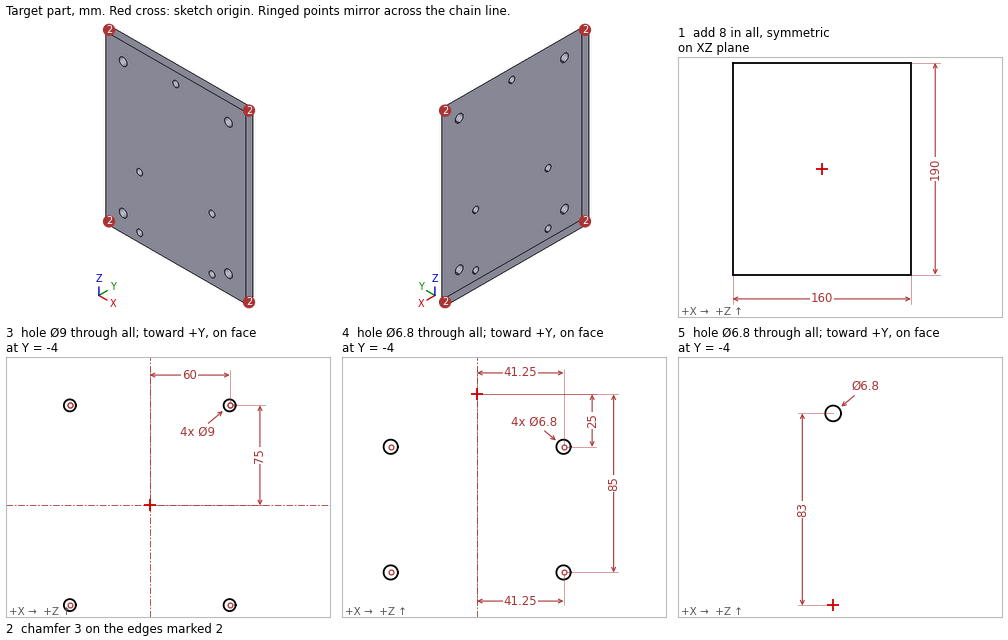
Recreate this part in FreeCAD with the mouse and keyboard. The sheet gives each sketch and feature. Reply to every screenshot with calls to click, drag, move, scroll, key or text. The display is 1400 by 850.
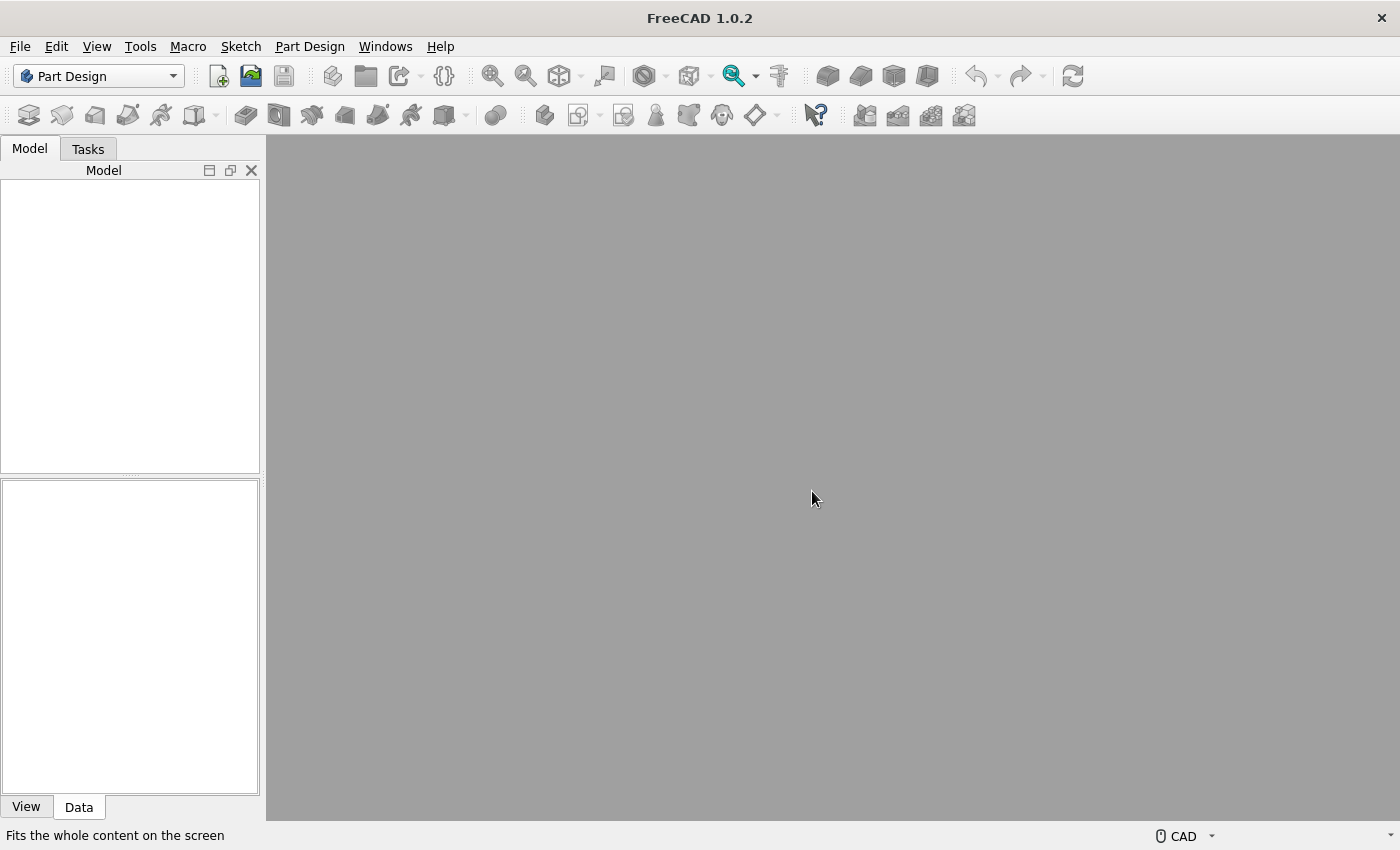
click(218, 76)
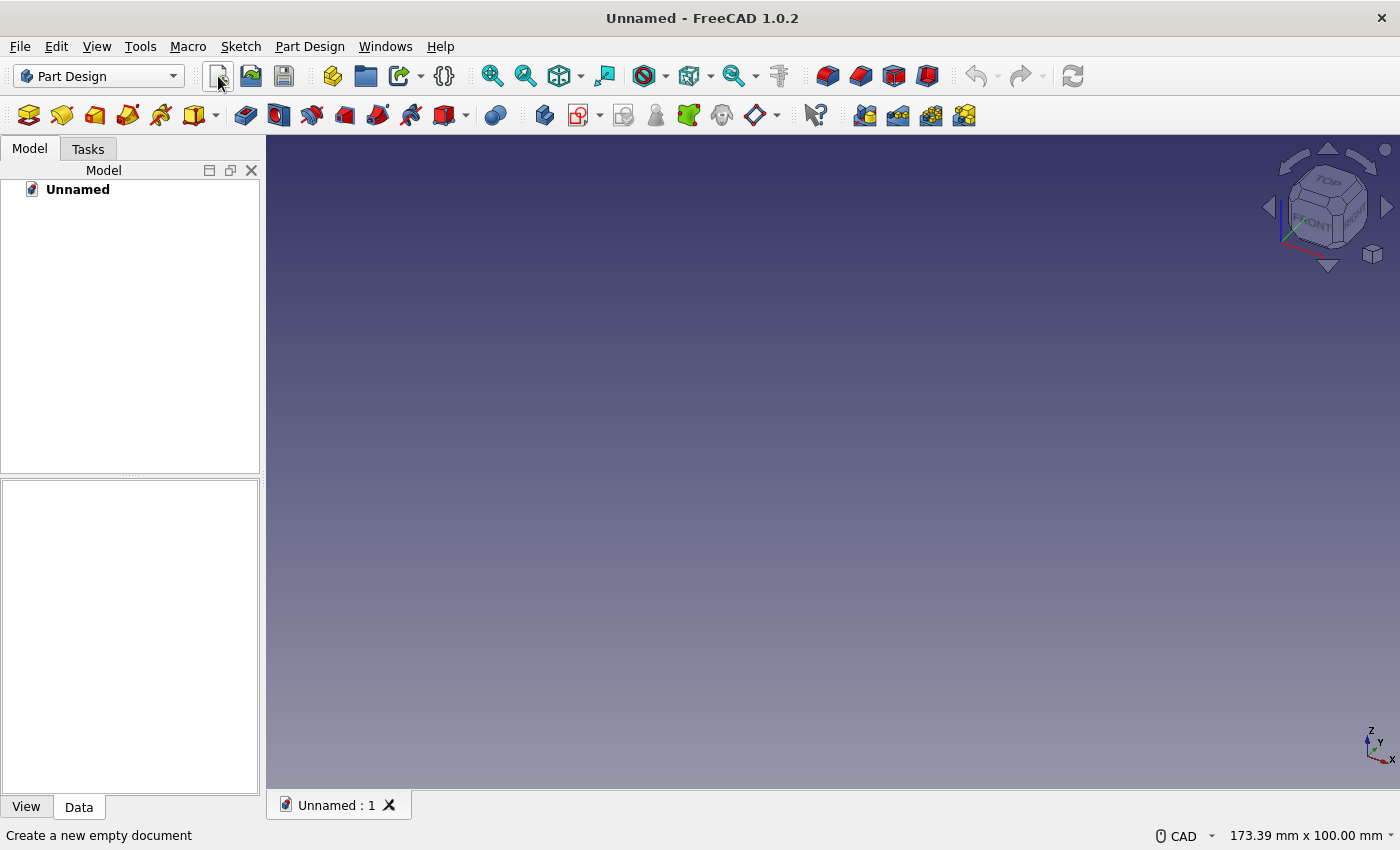
click(578, 116)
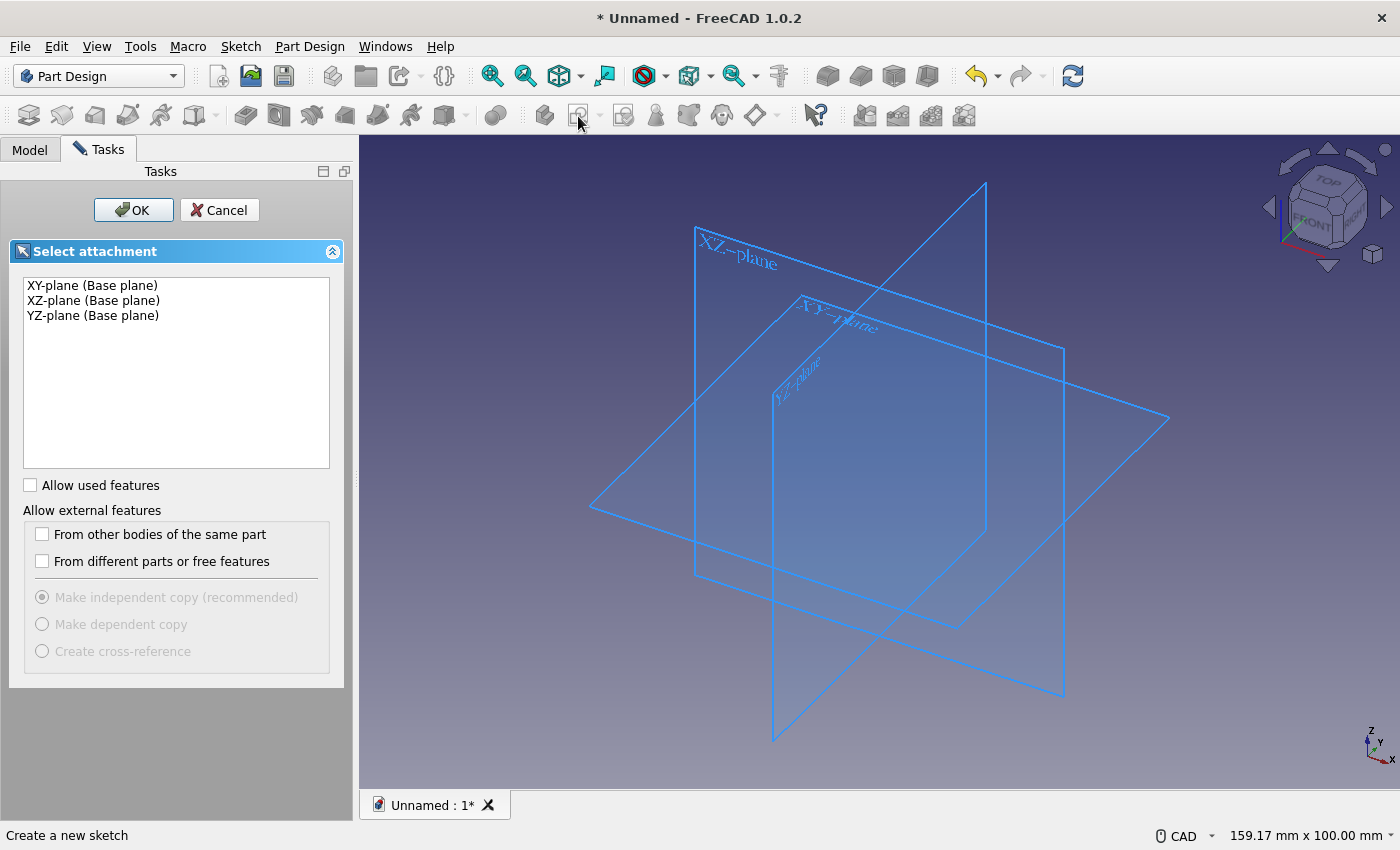
click(84, 300)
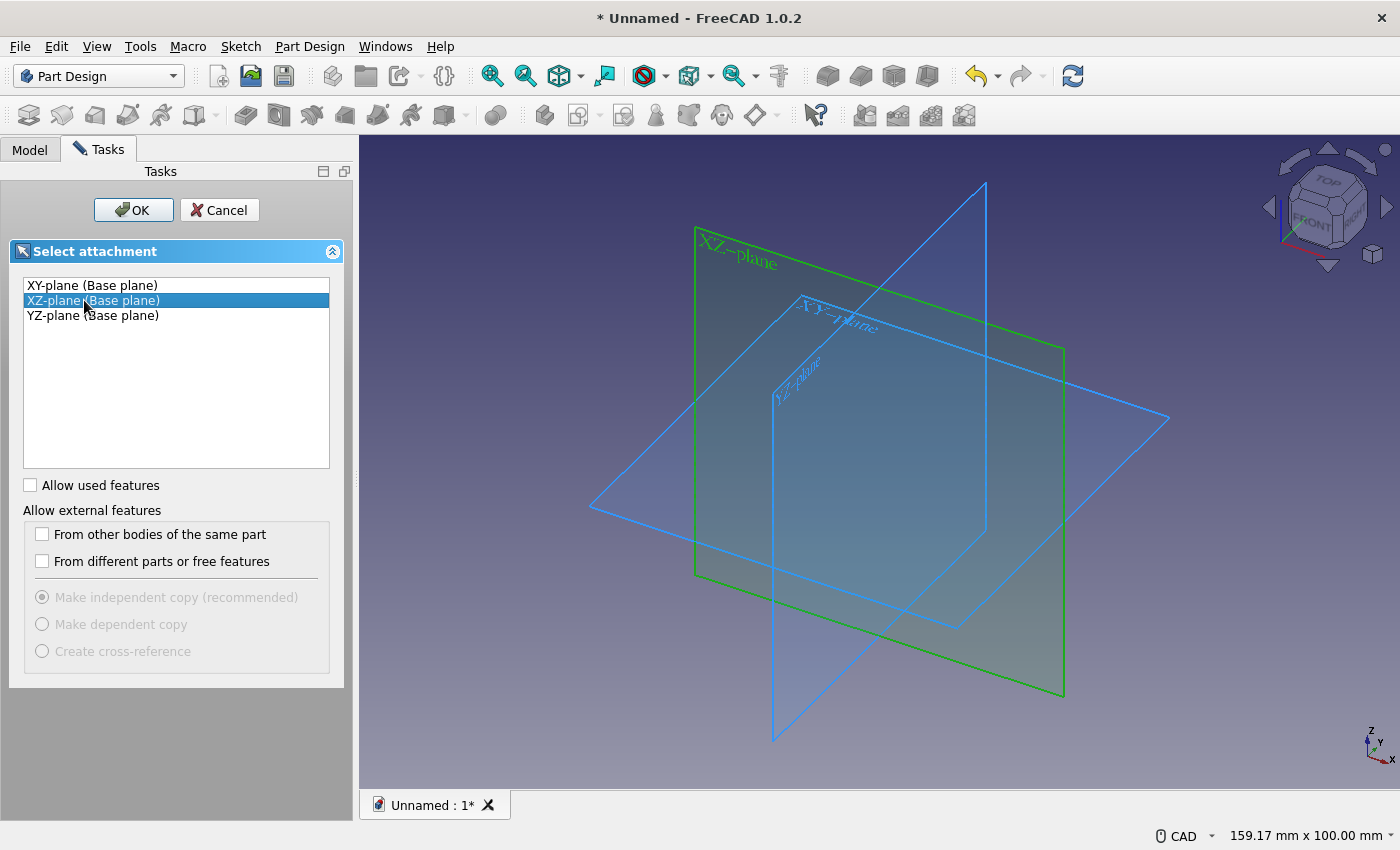
click(134, 210)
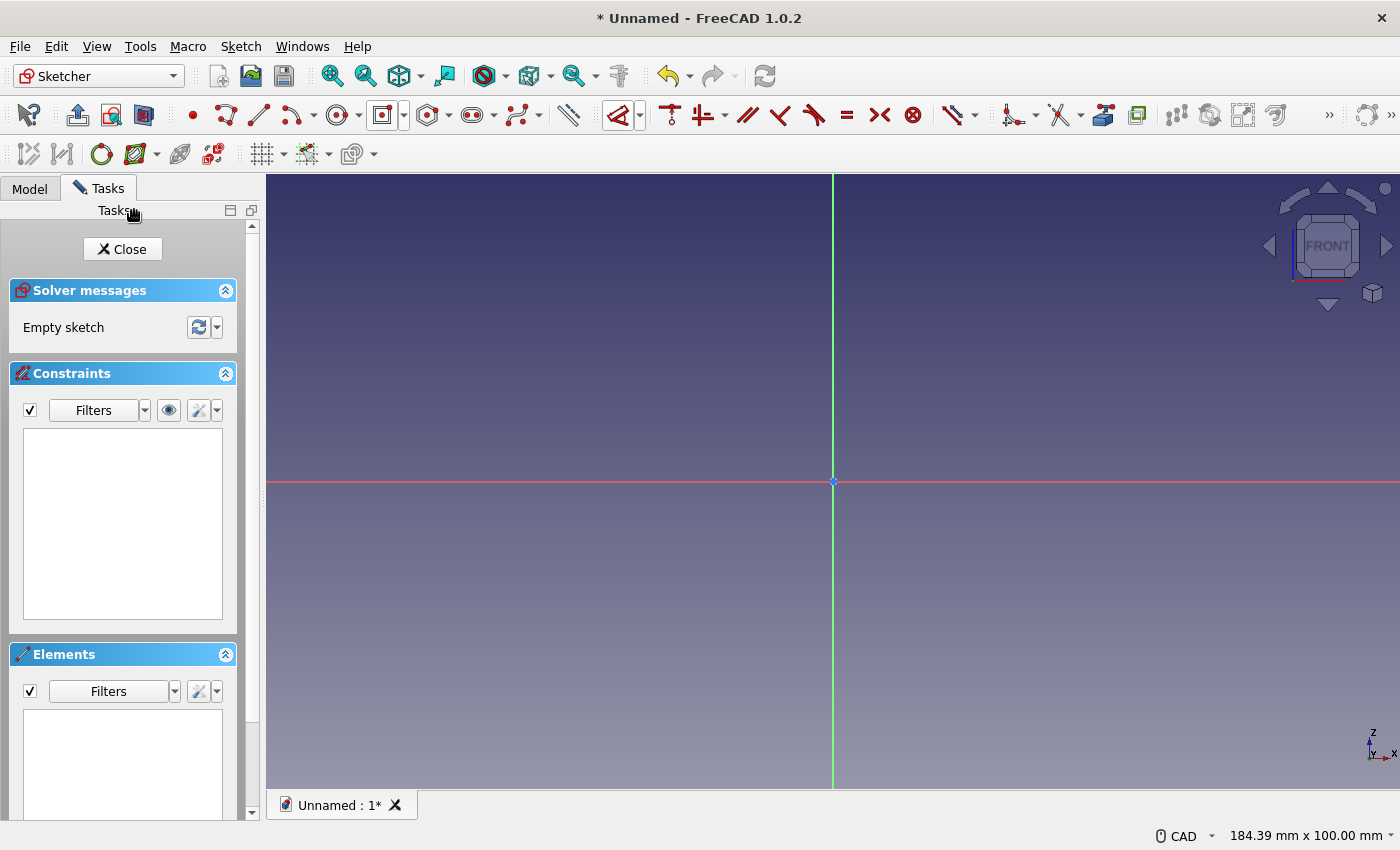
scroll(725, 482, down, 5)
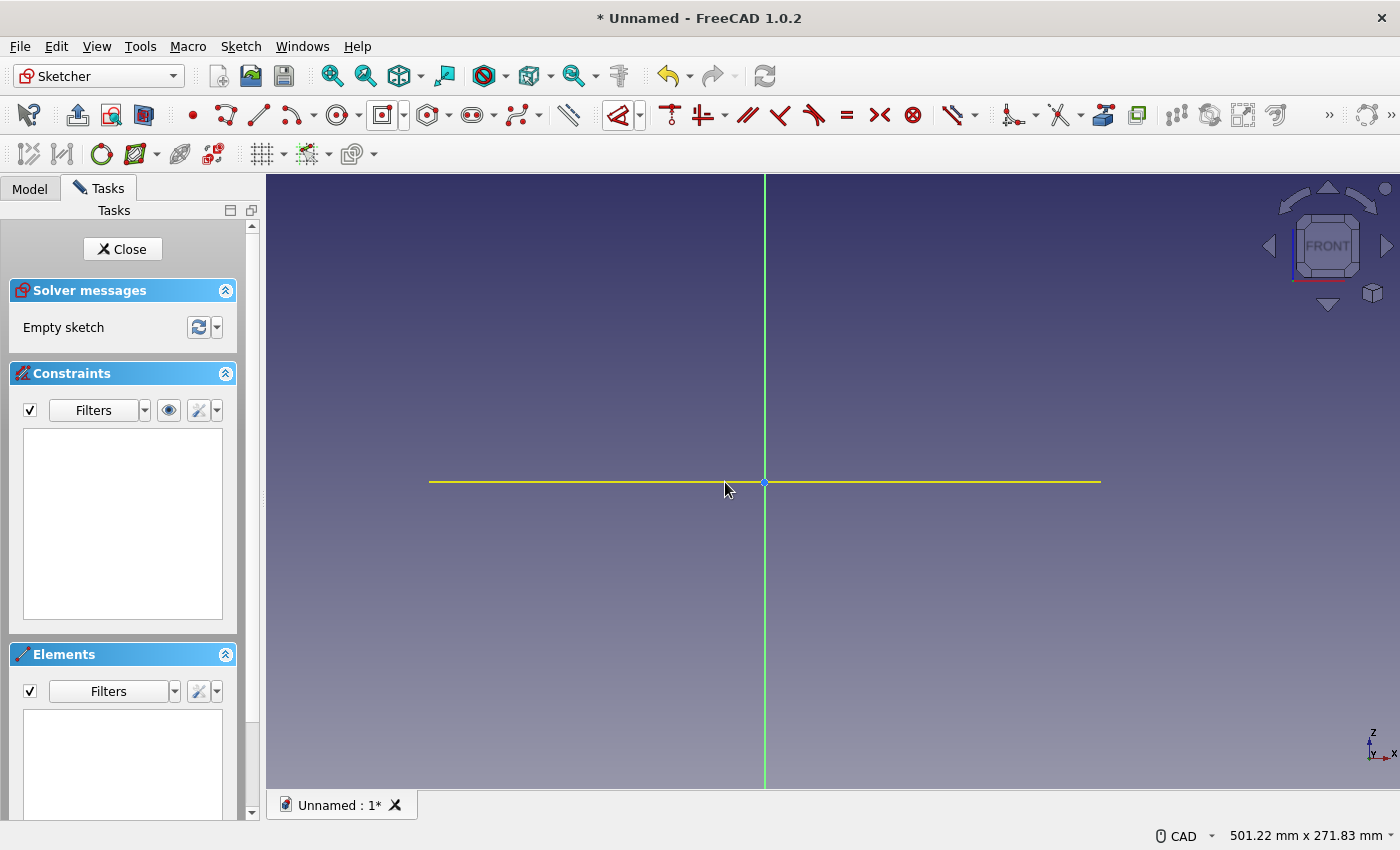
click(382, 116)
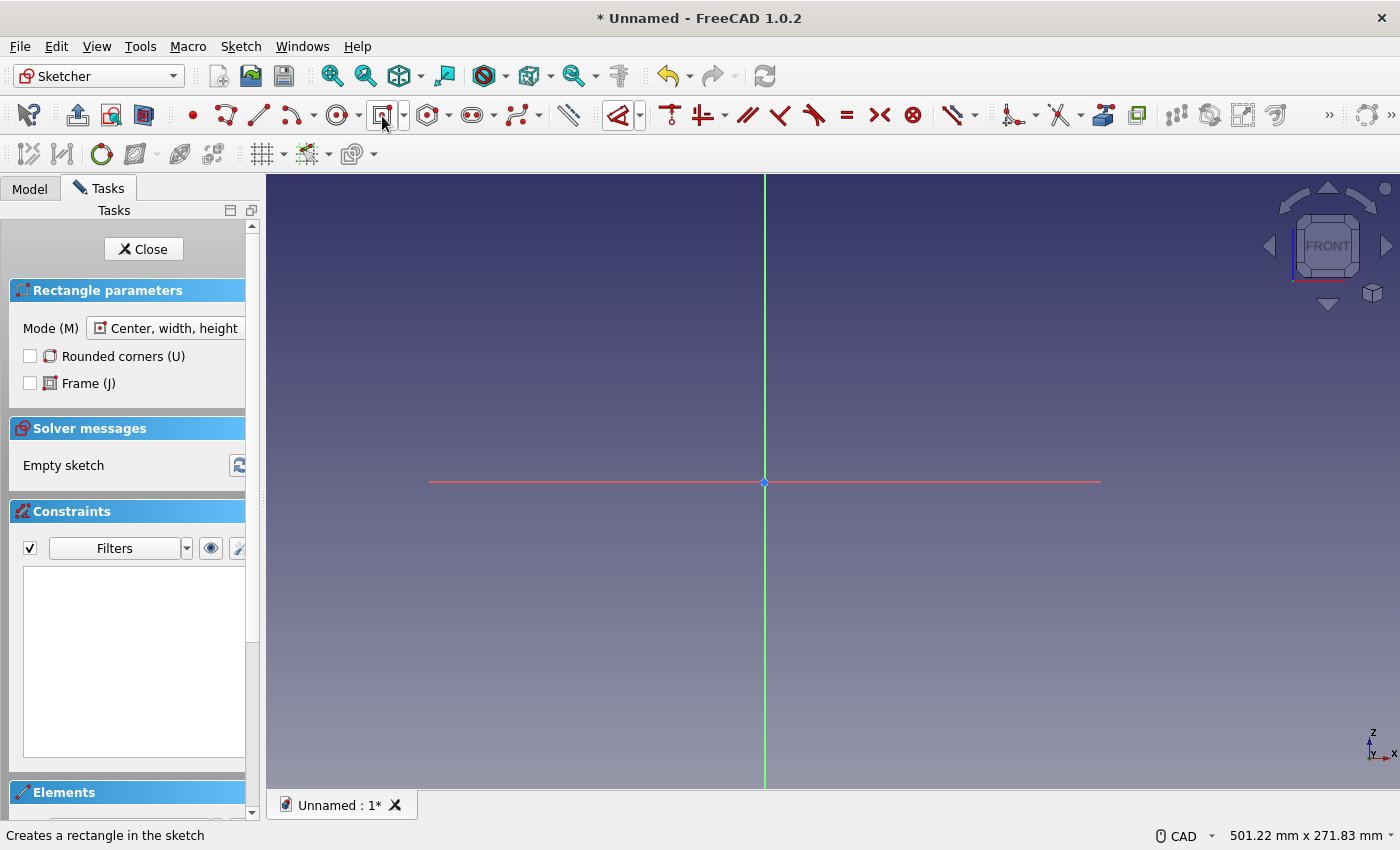
click(765, 482)
click(946, 267)
key(Escape)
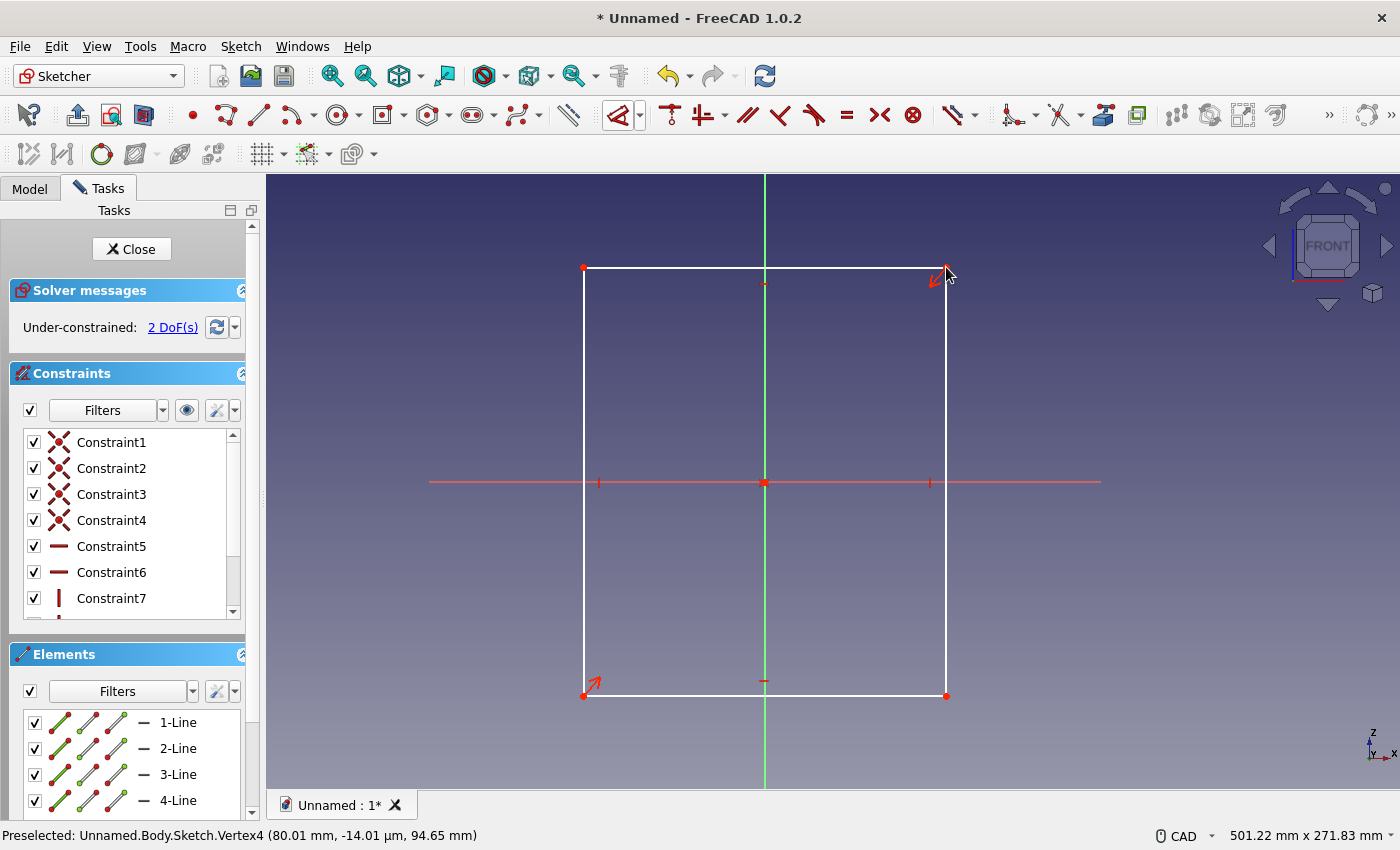
click(618, 116)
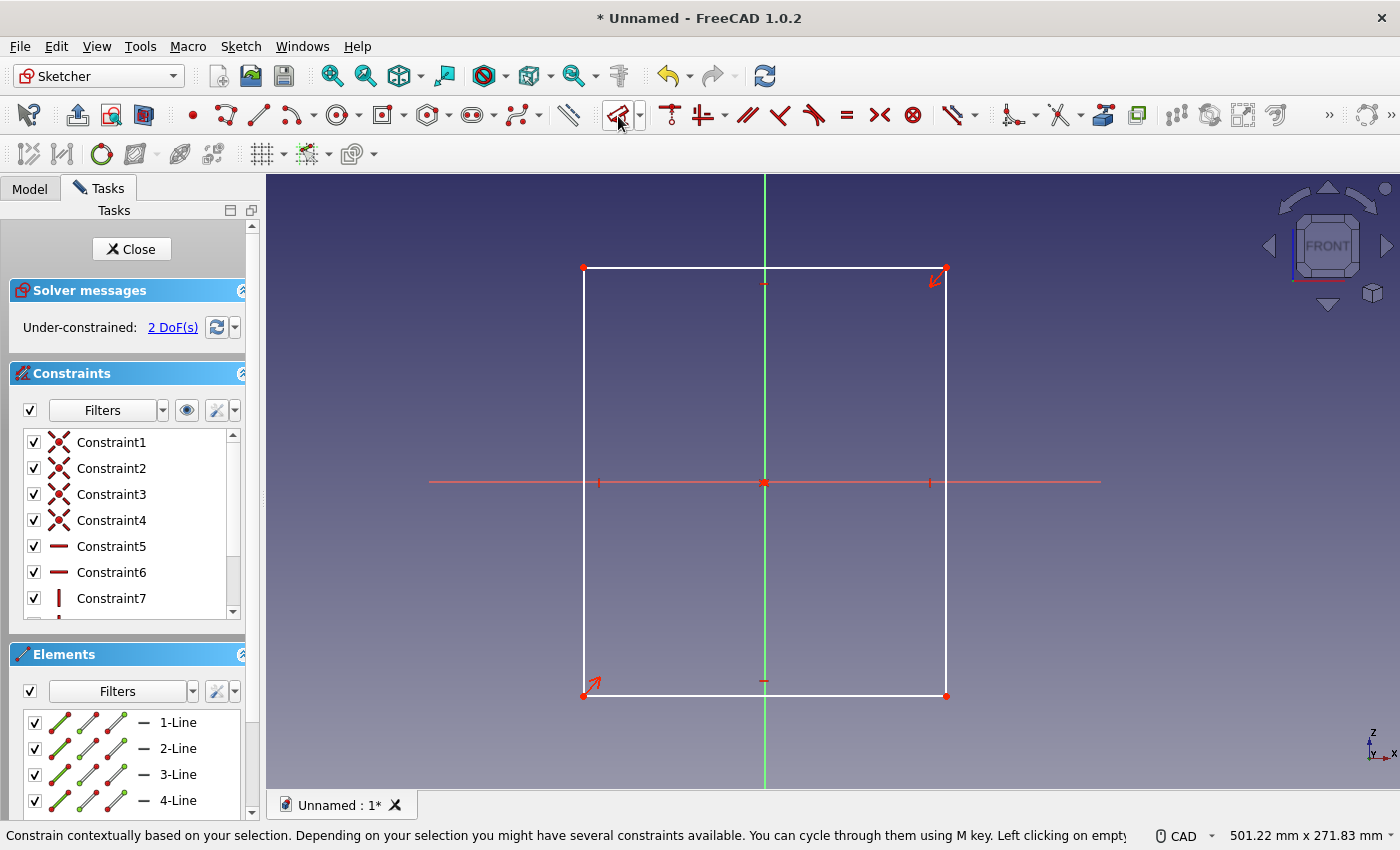
click(693, 696)
click(682, 730)